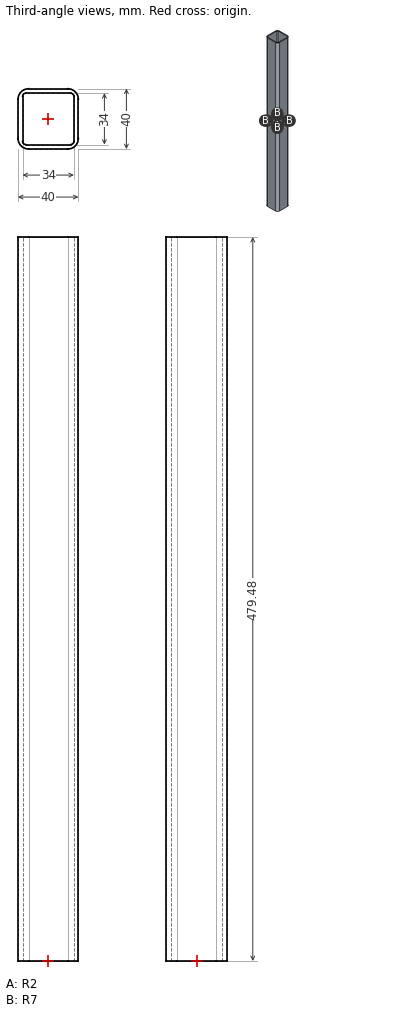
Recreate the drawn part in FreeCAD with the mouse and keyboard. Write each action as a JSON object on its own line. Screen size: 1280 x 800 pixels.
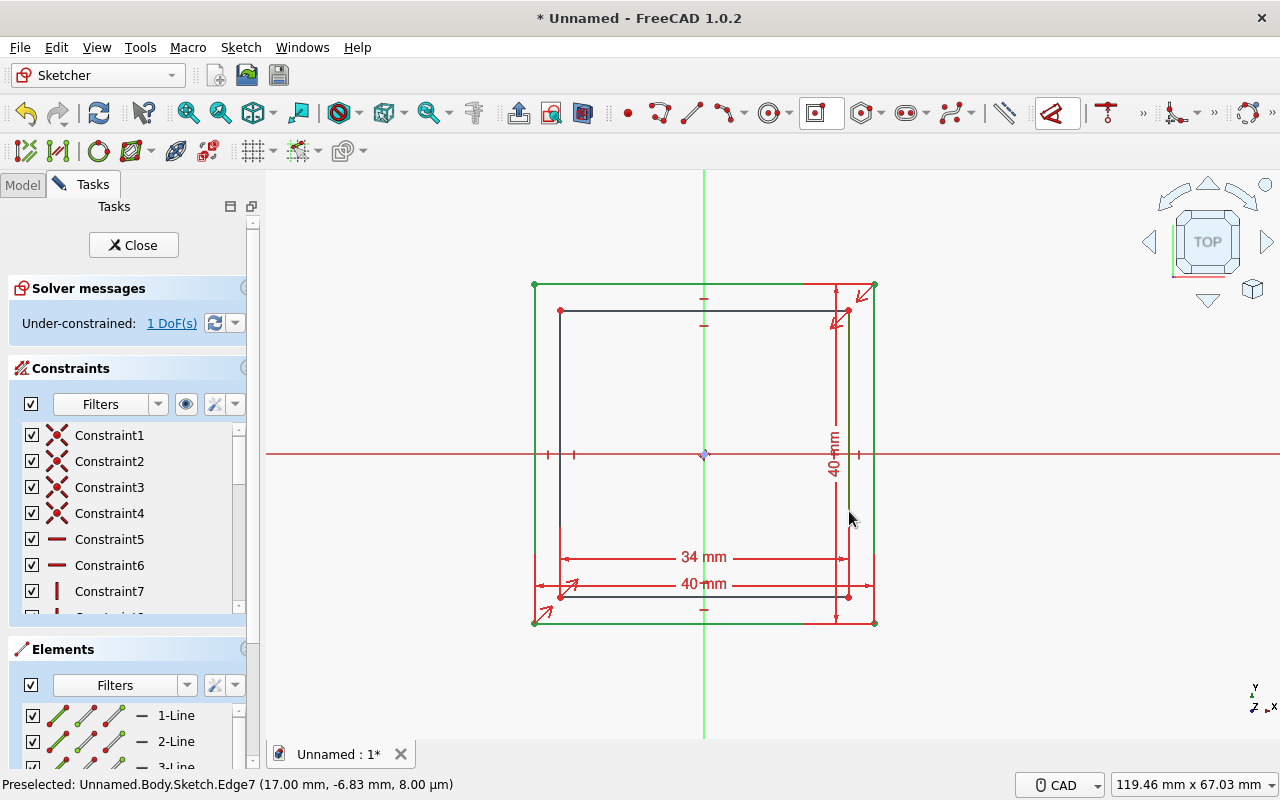
{"action": "key", "text": "i"}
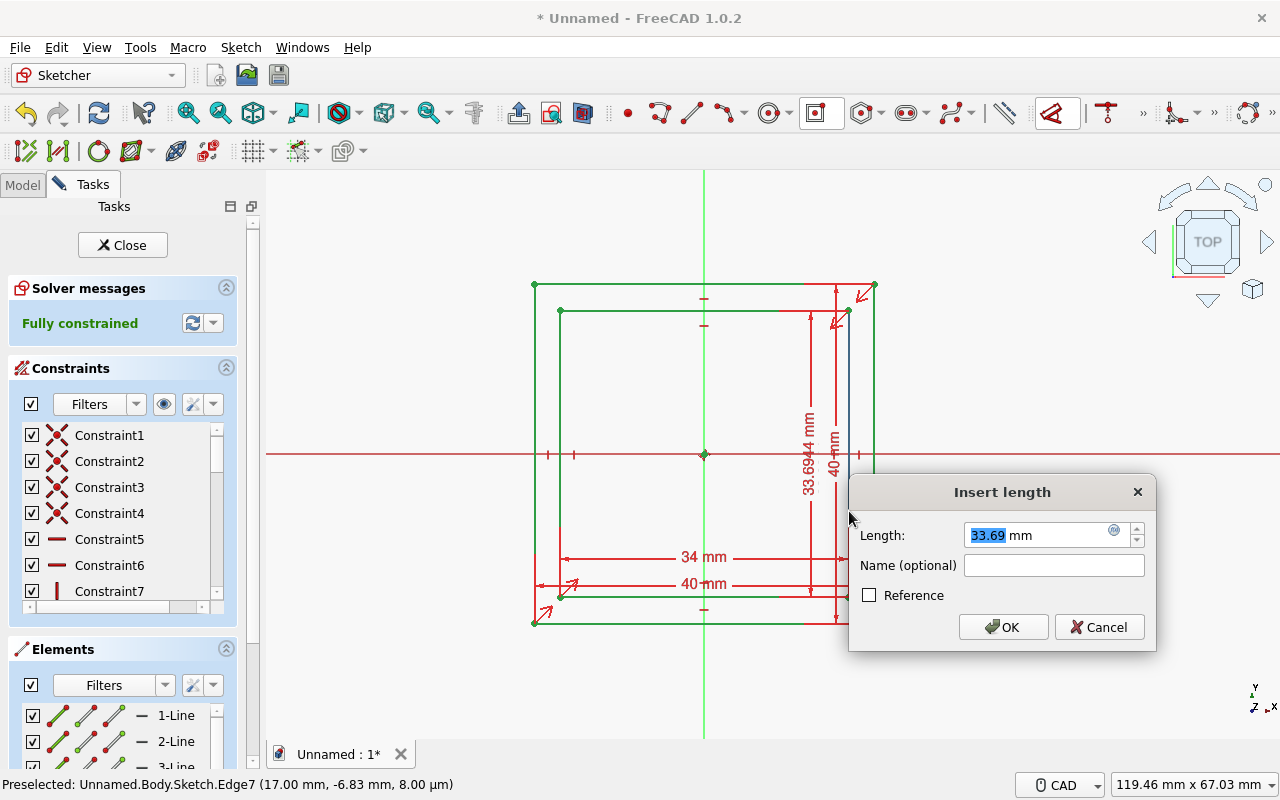
{"action": "type", "text": "34"}
{"action": "key", "text": "Return"}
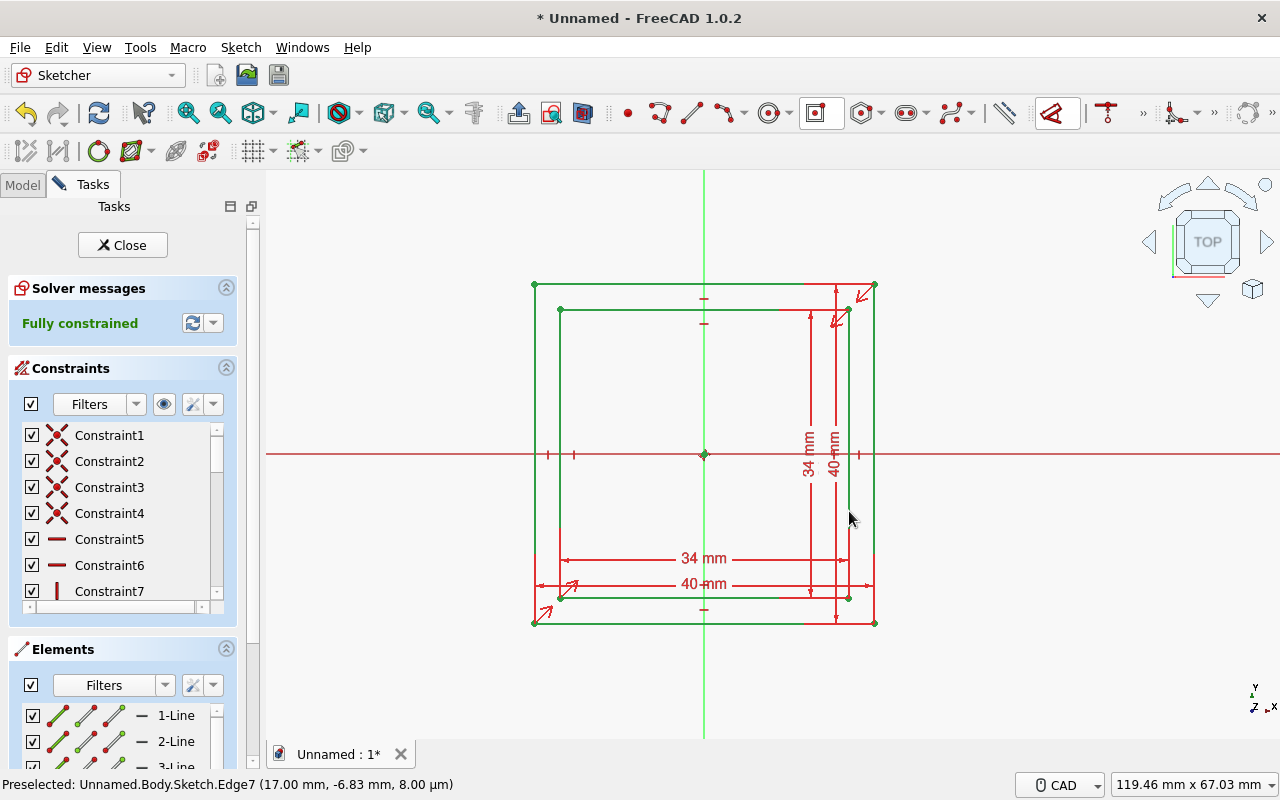
{"action": "left_click", "coordinate": [123, 245]}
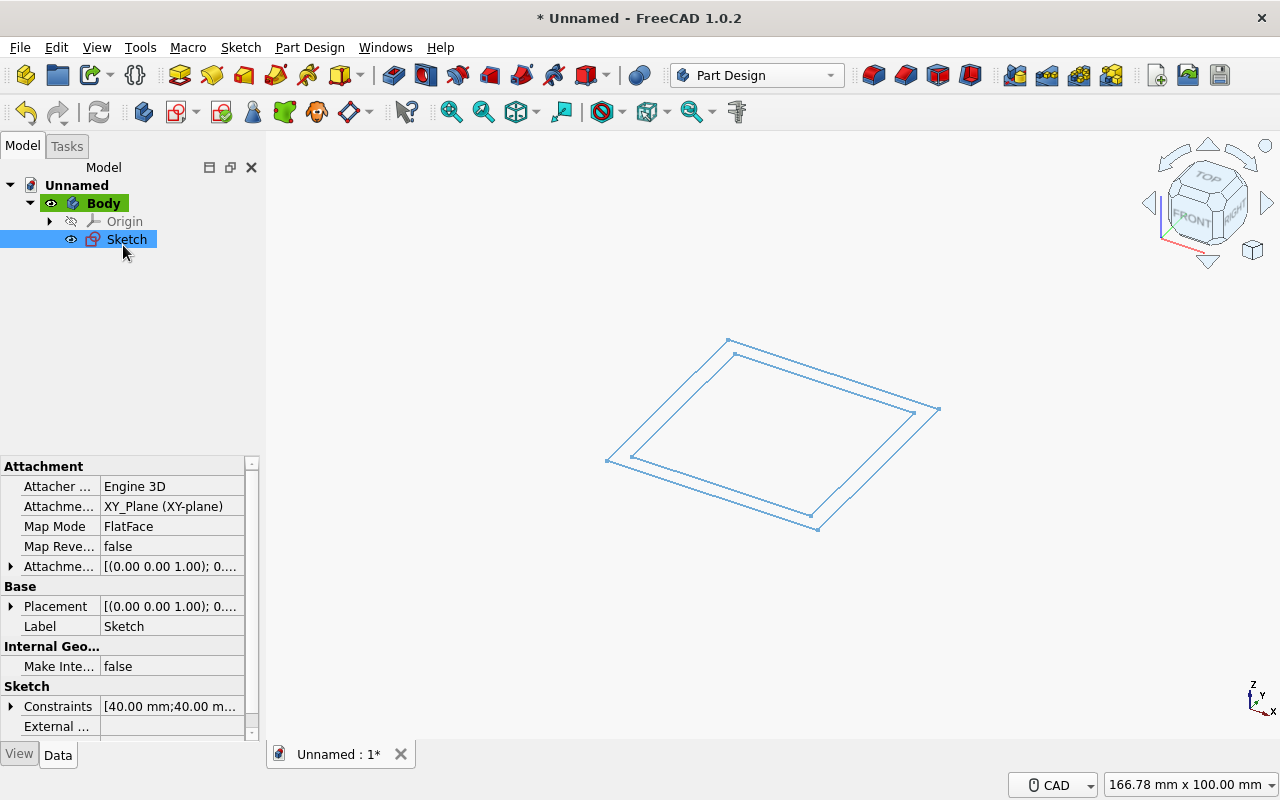
{"action": "left_click", "coordinate": [180, 76]}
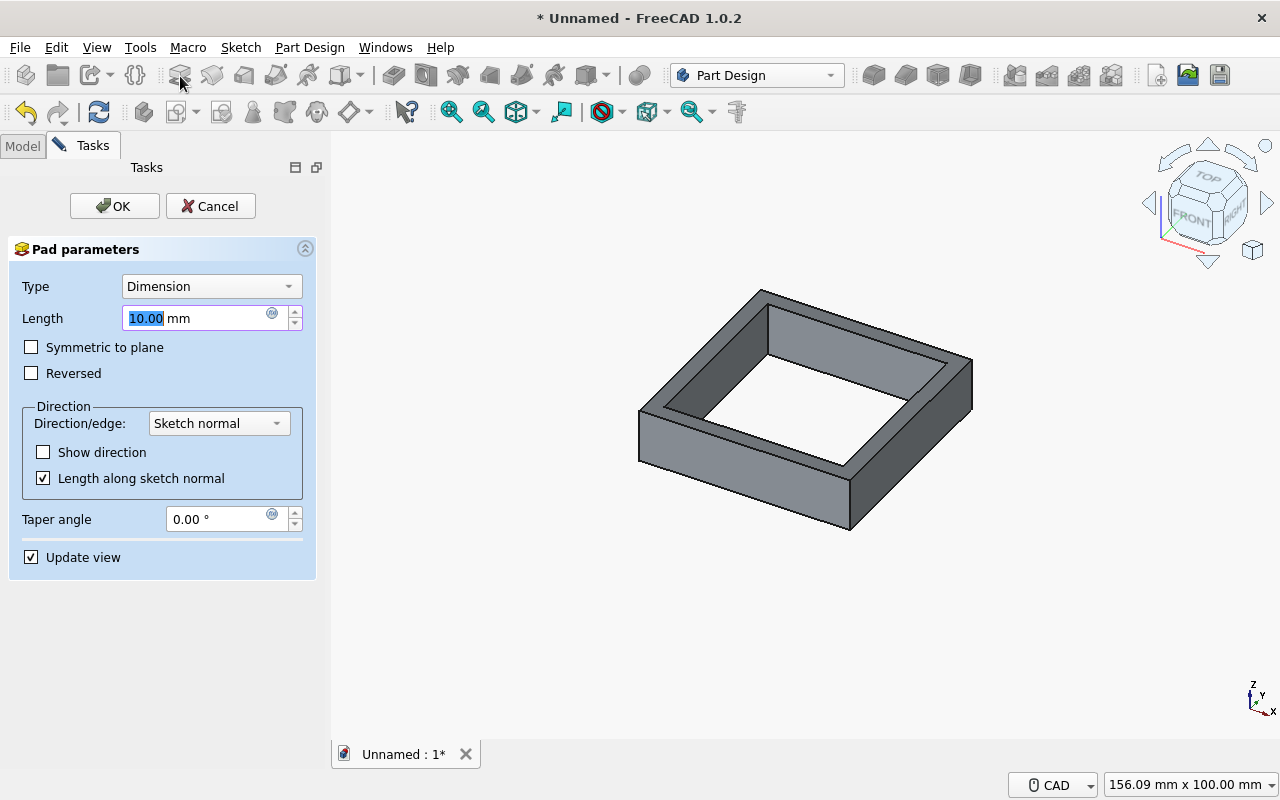
{"action": "type", "text": "479.48"}
{"action": "key", "text": "Tab"}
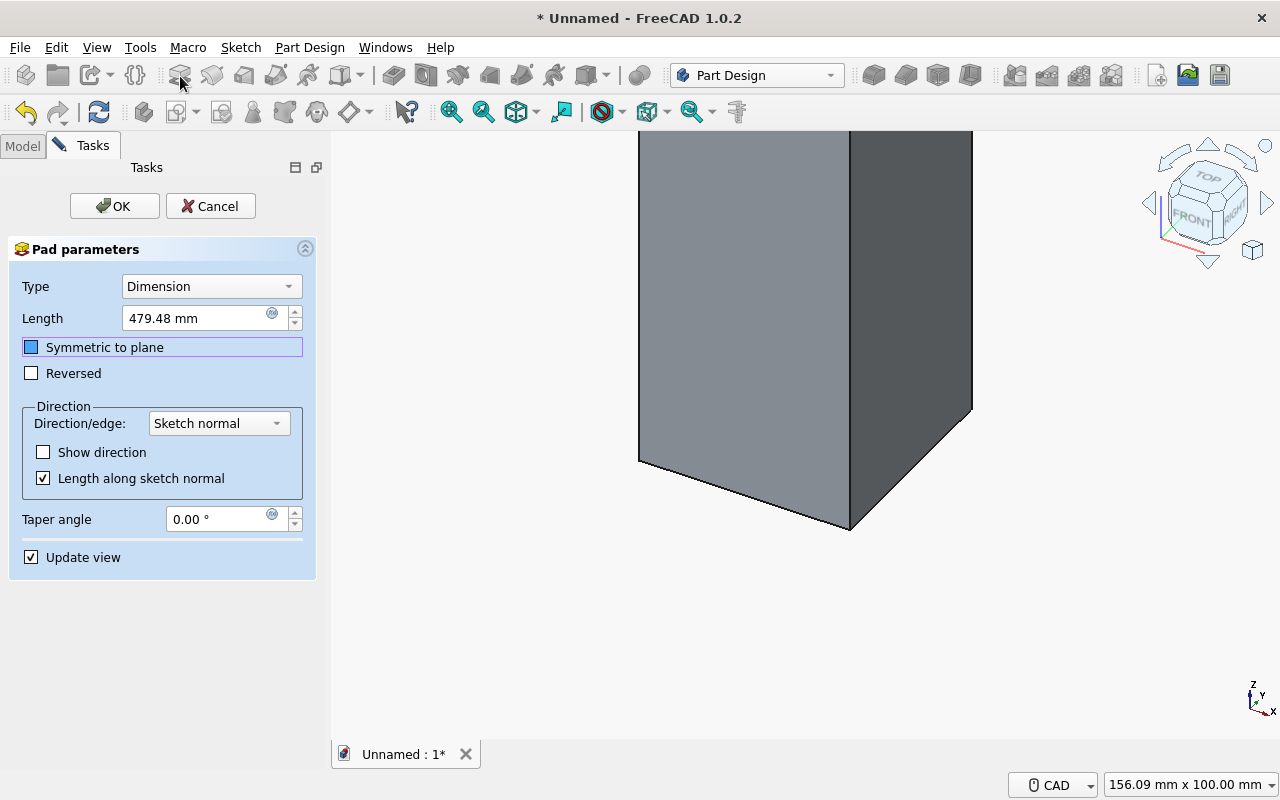
{"action": "left_click", "coordinate": [115, 206]}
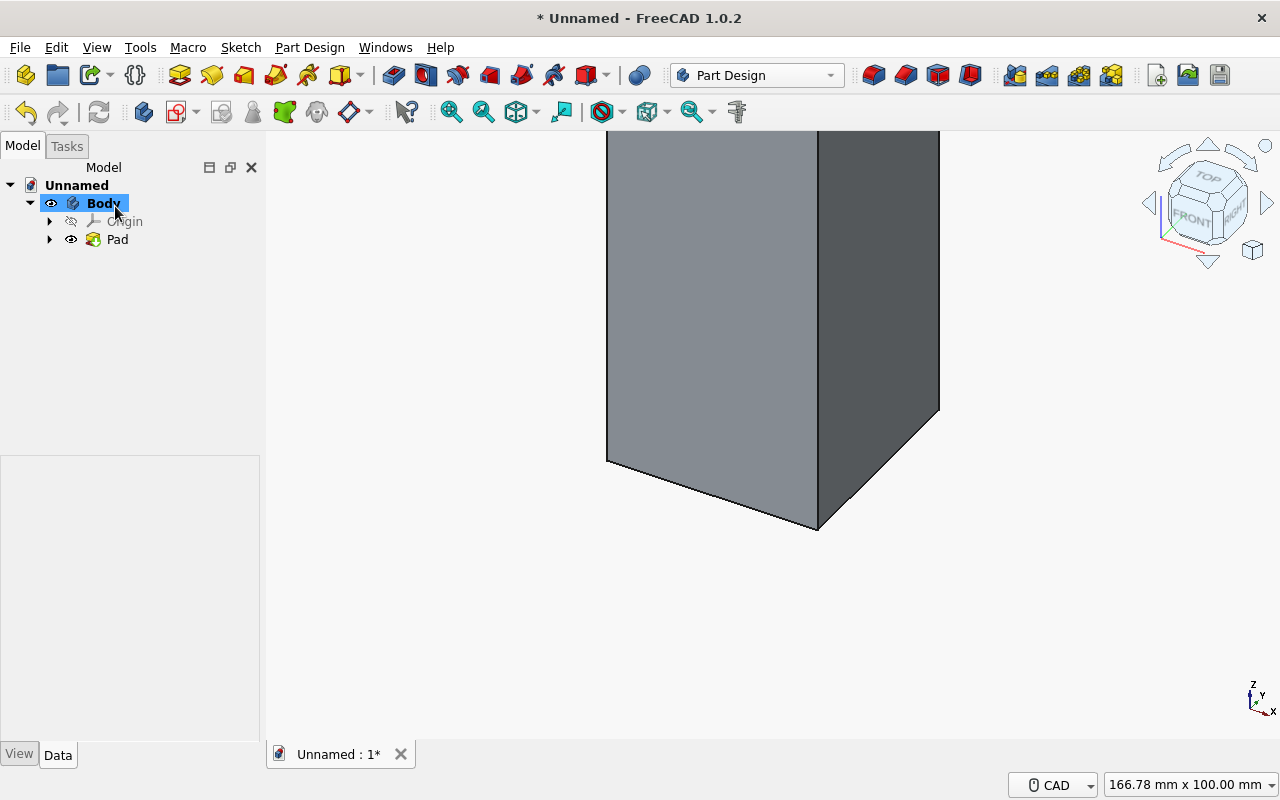
{"action": "key", "text": "v f"}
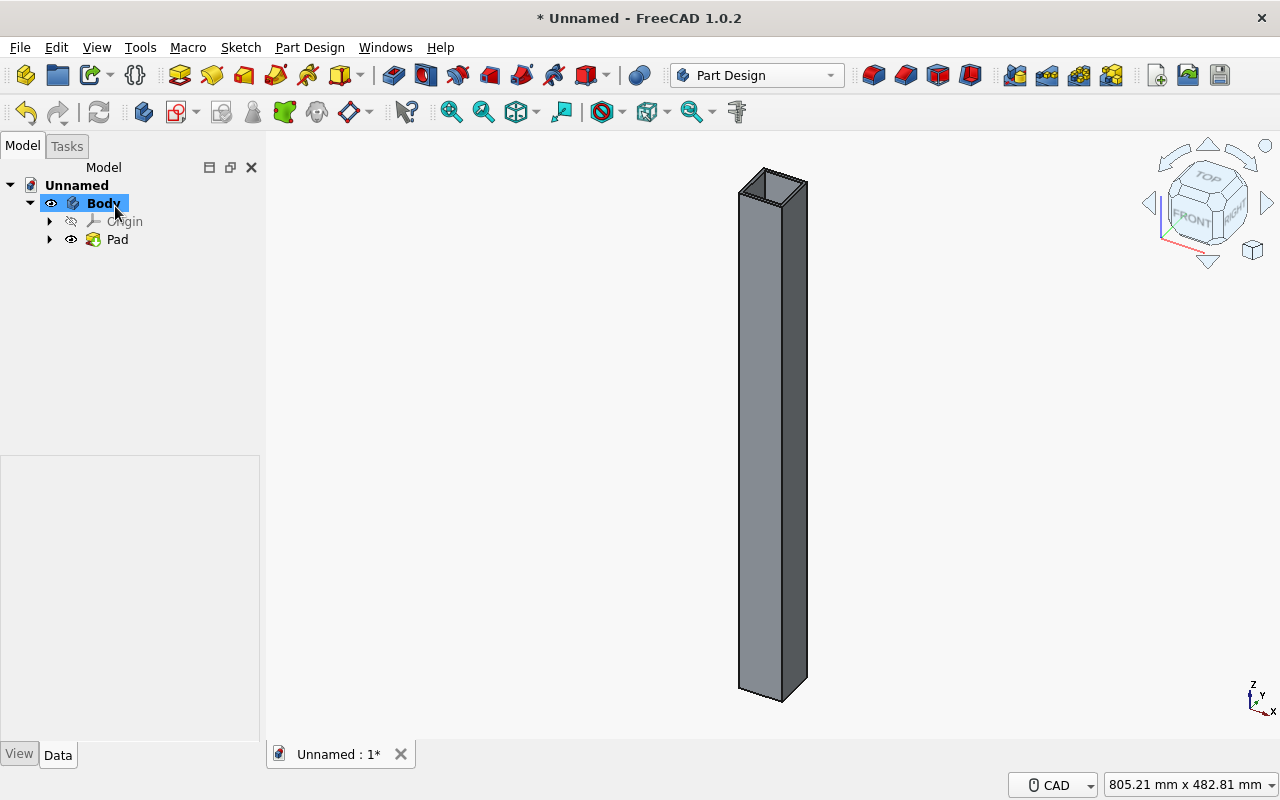
{"action": "key", "text": "0"}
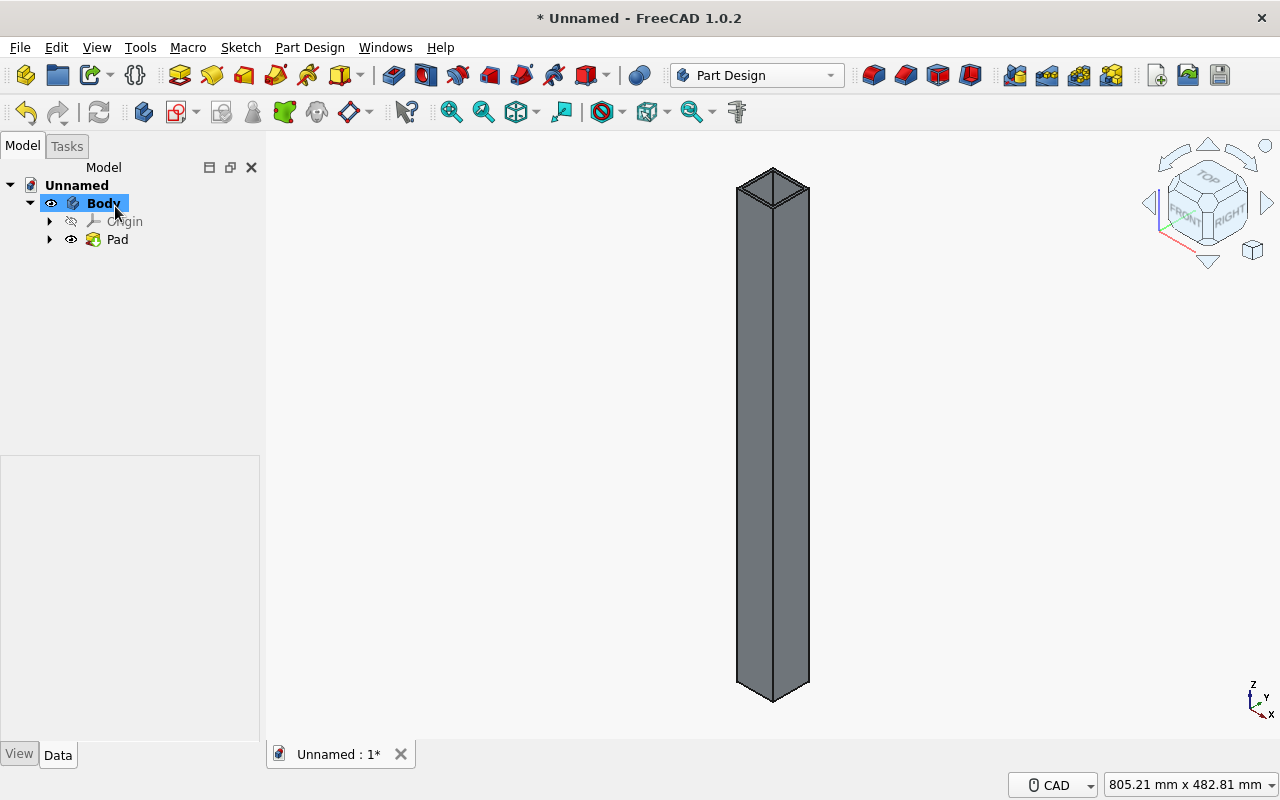
{"action": "key", "text": "2"}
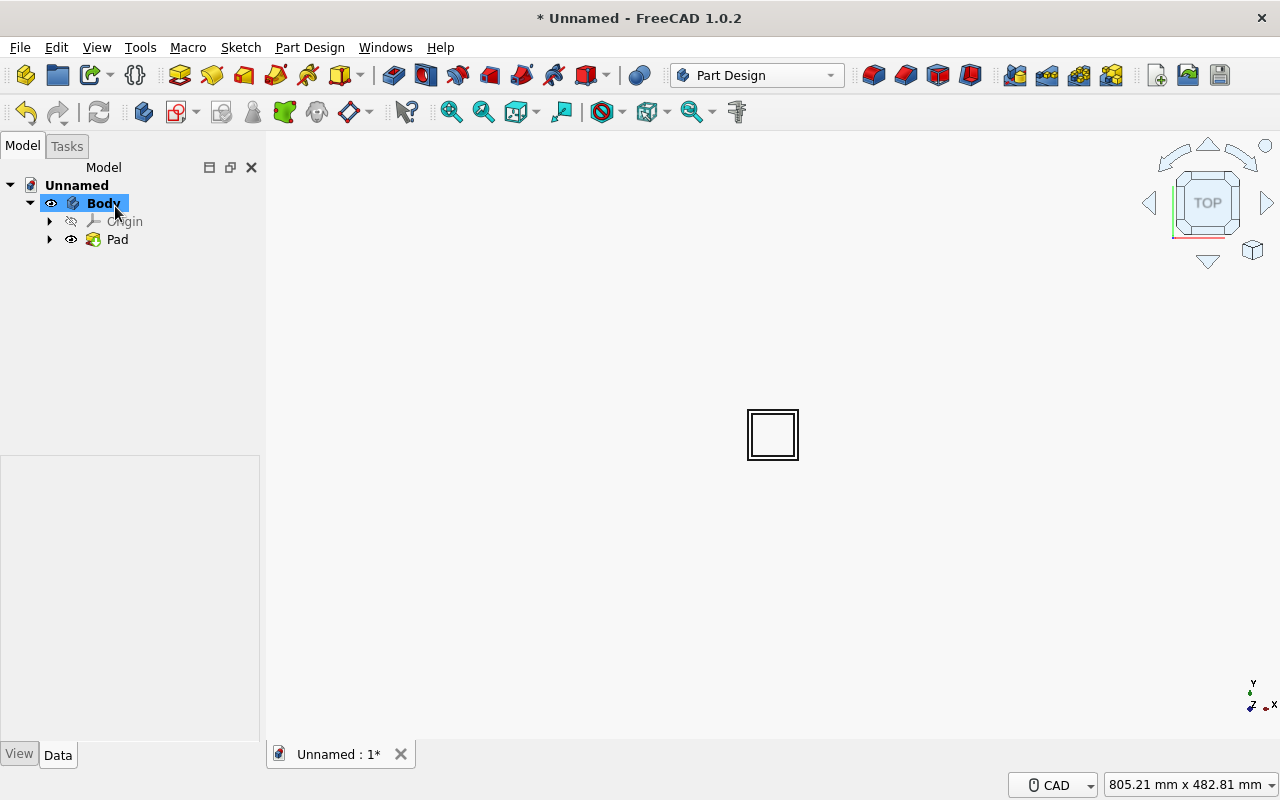
{"action": "left_click", "coordinate": [452, 112]}